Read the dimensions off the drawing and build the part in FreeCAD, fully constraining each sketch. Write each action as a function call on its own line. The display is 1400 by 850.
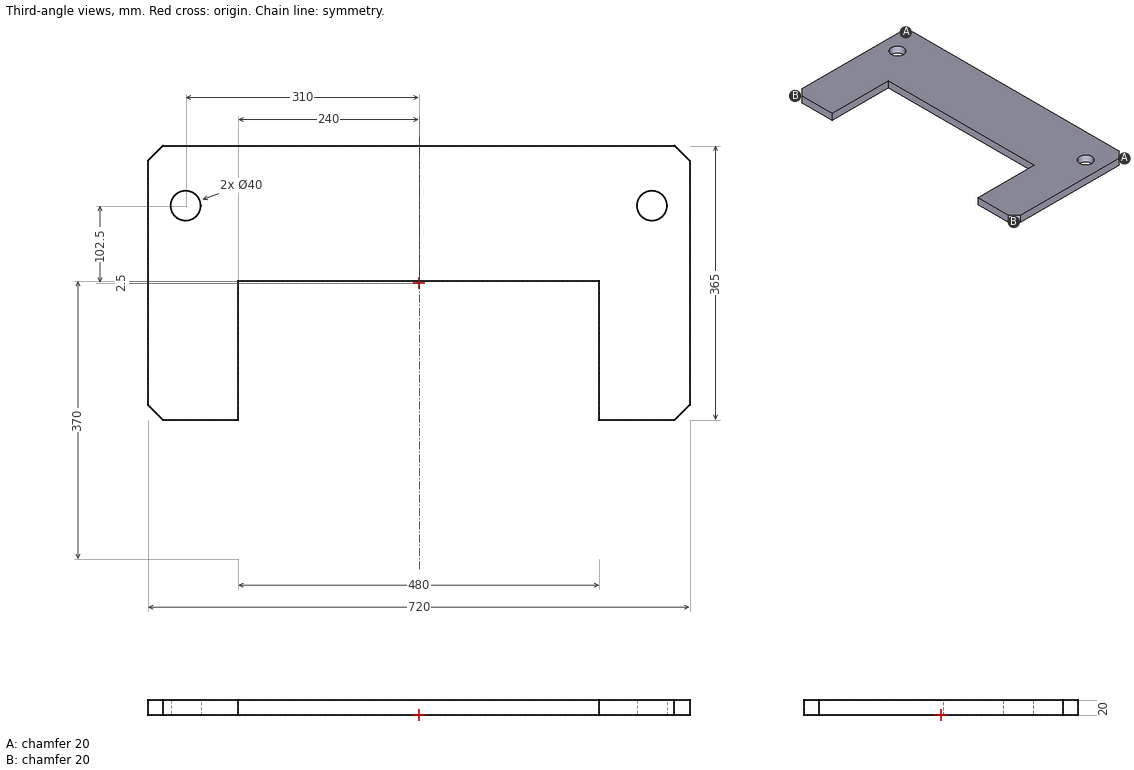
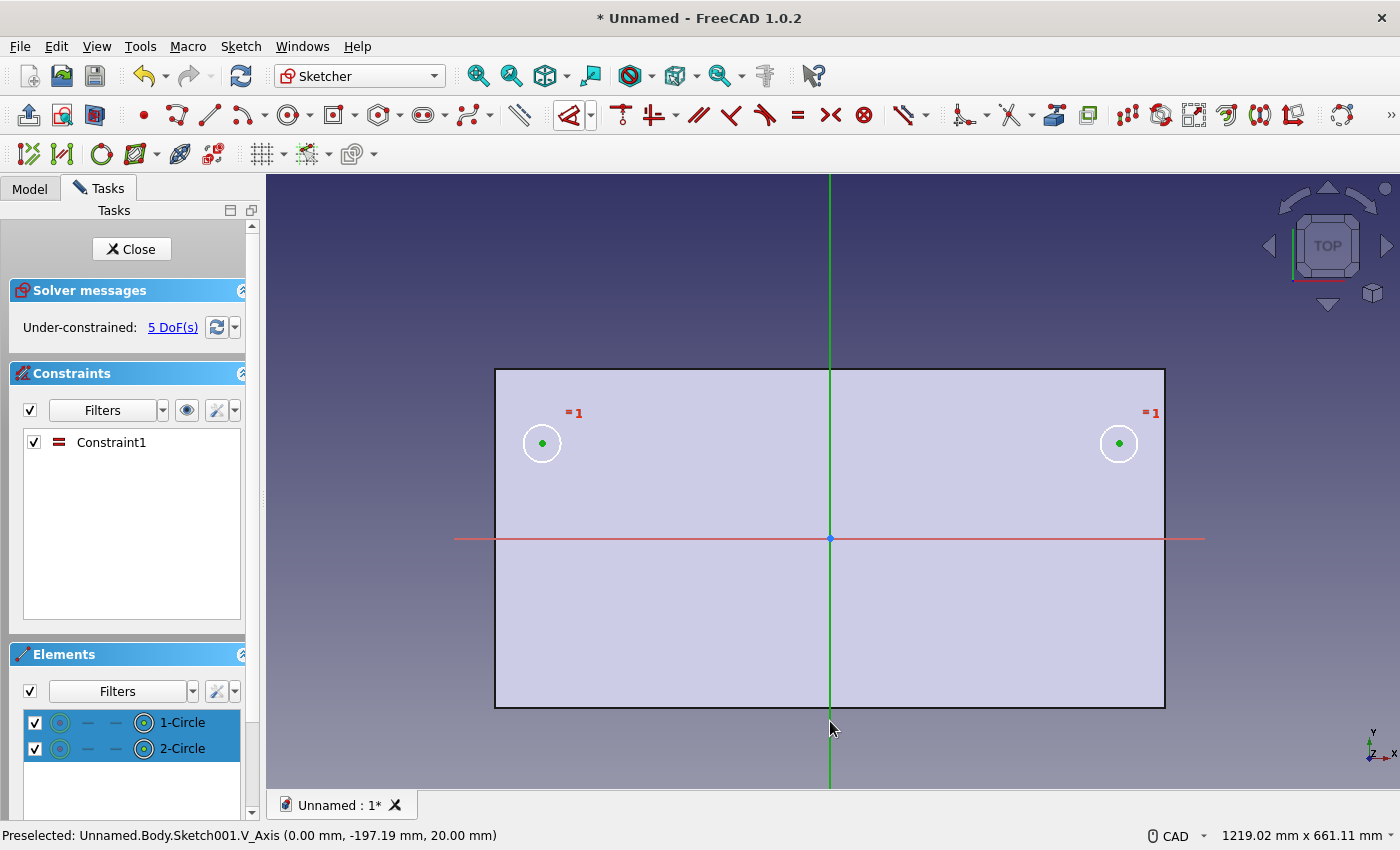
key(s)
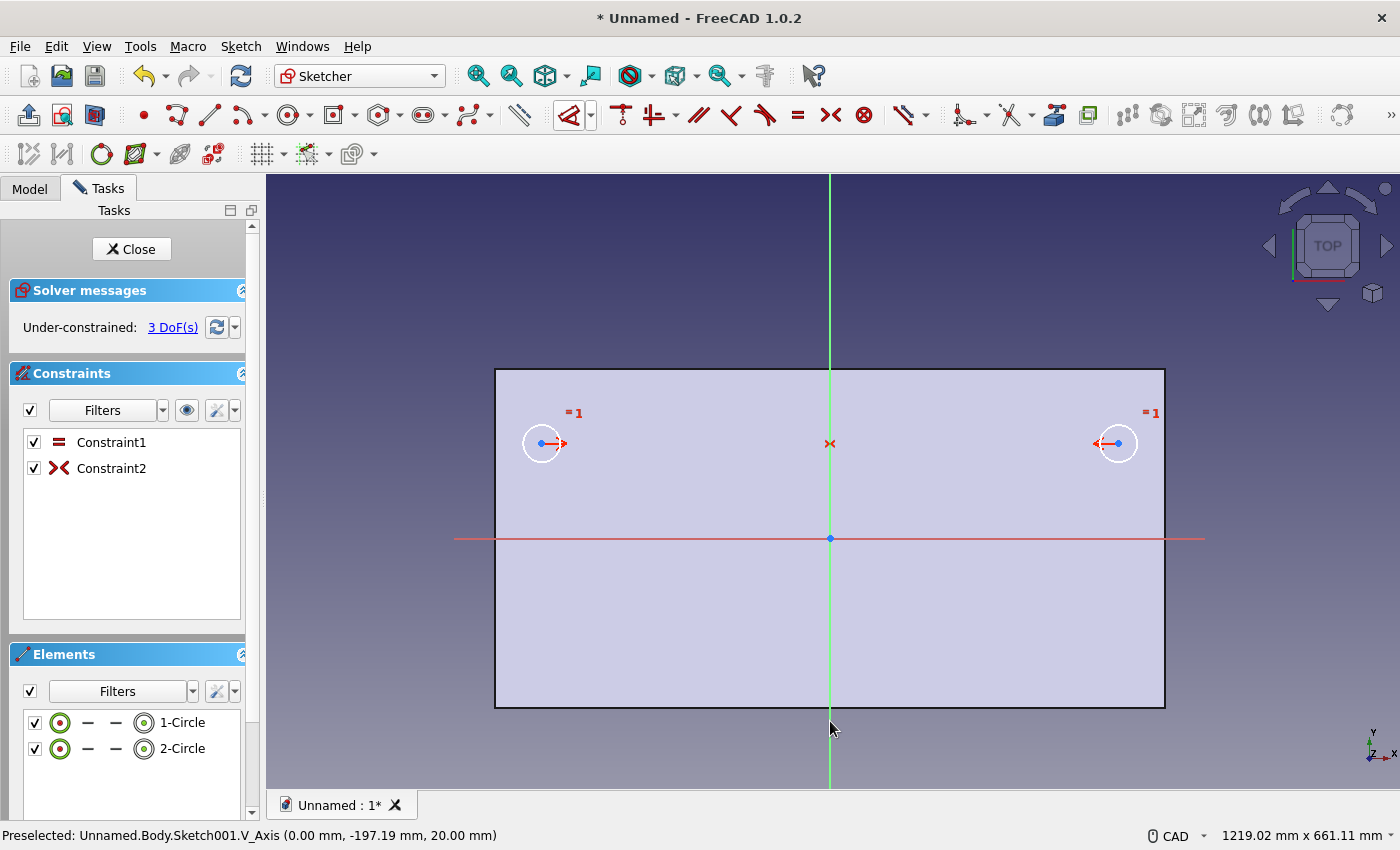
click(555, 431)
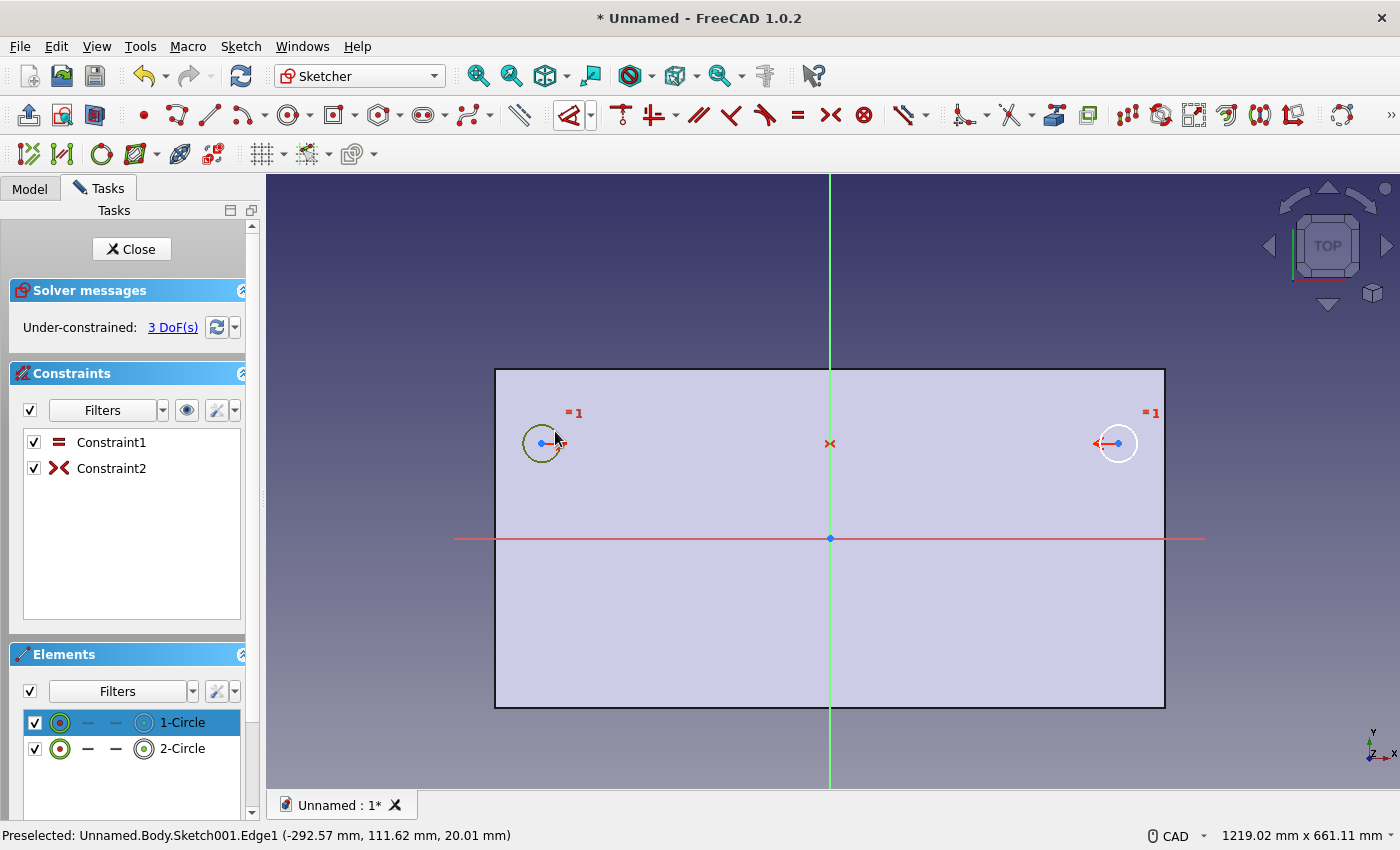
key(k)
key(o)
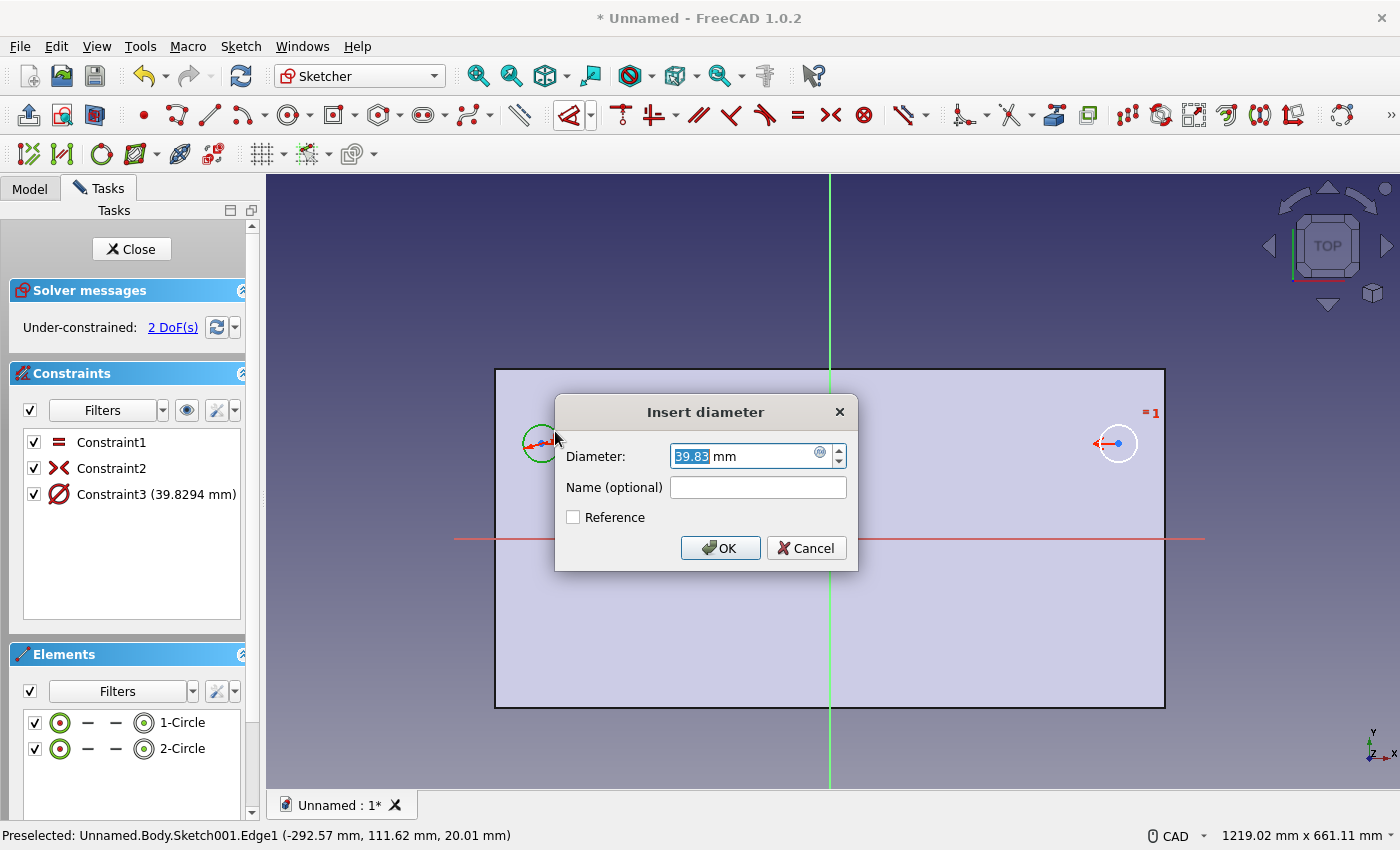
text(40)
key(Return)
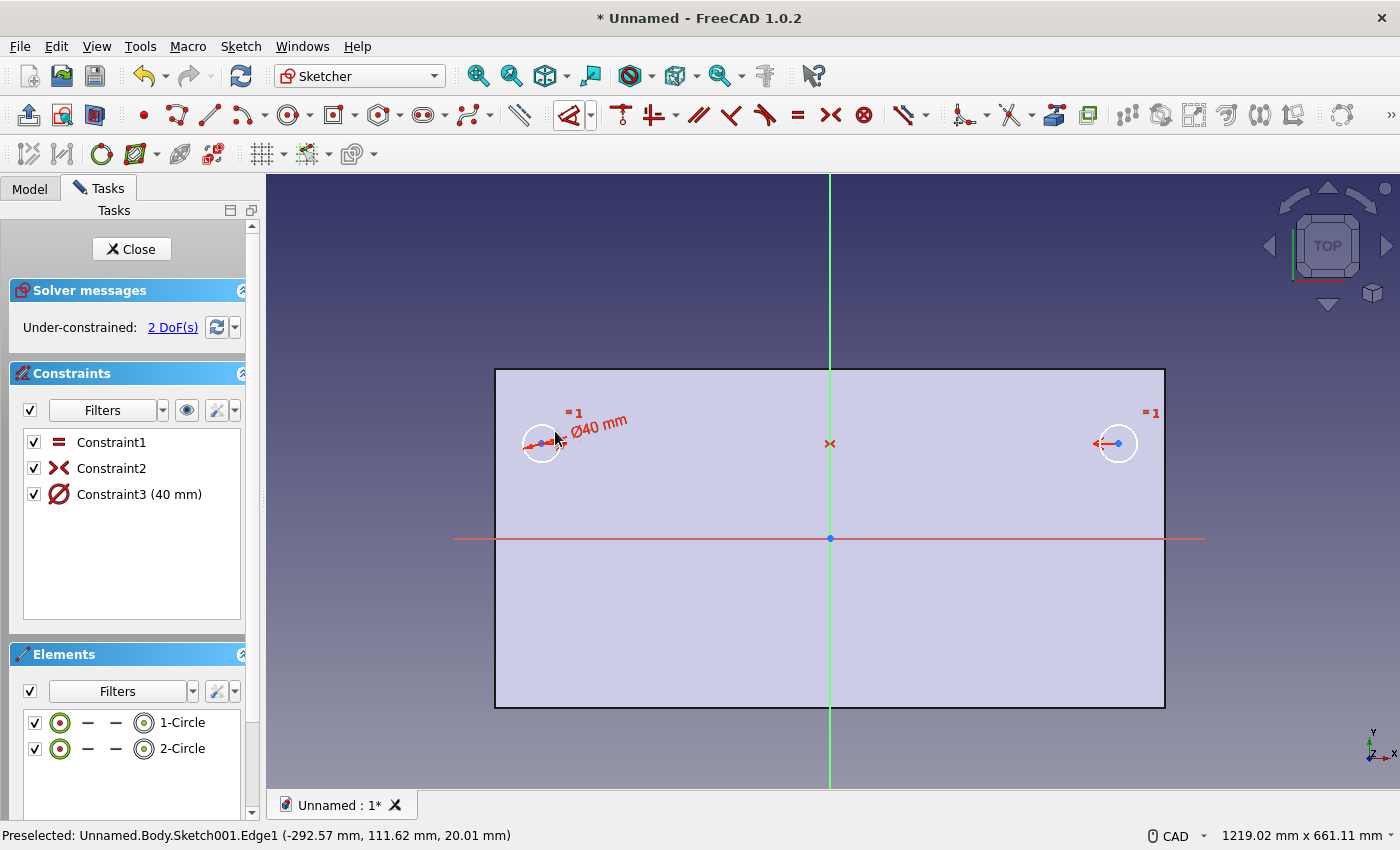
click(542, 444)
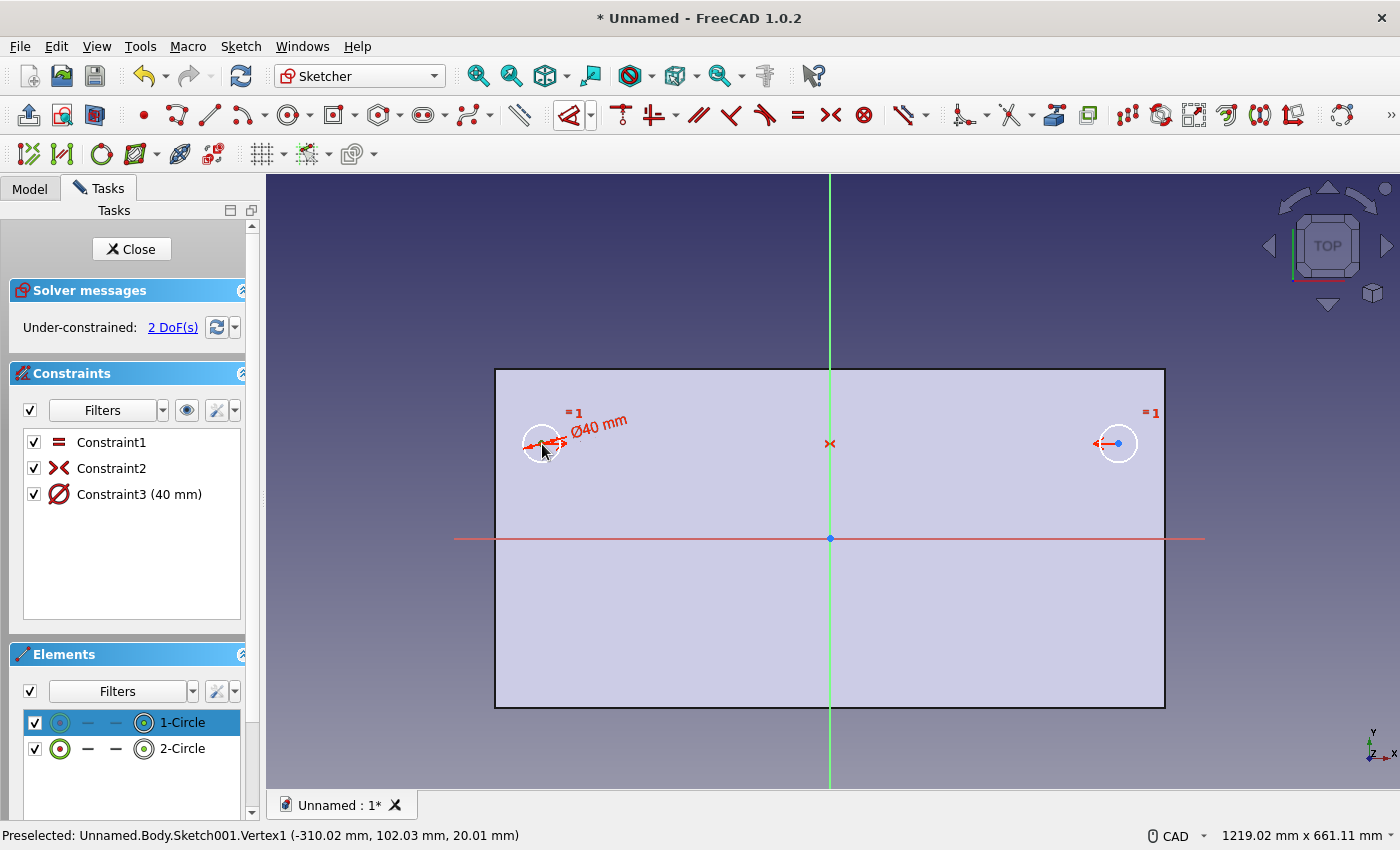
key(l)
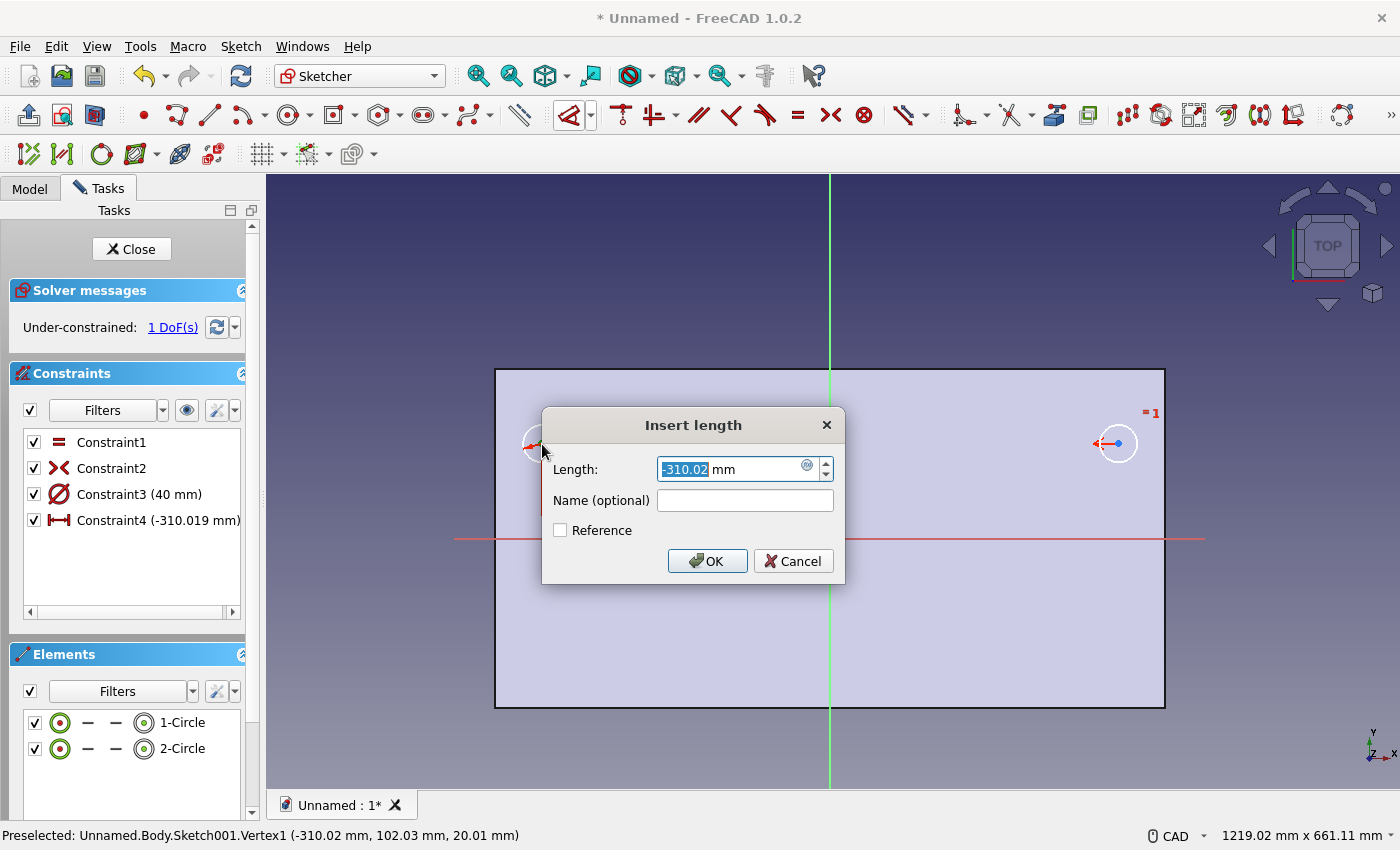
text(-310)
key(Return)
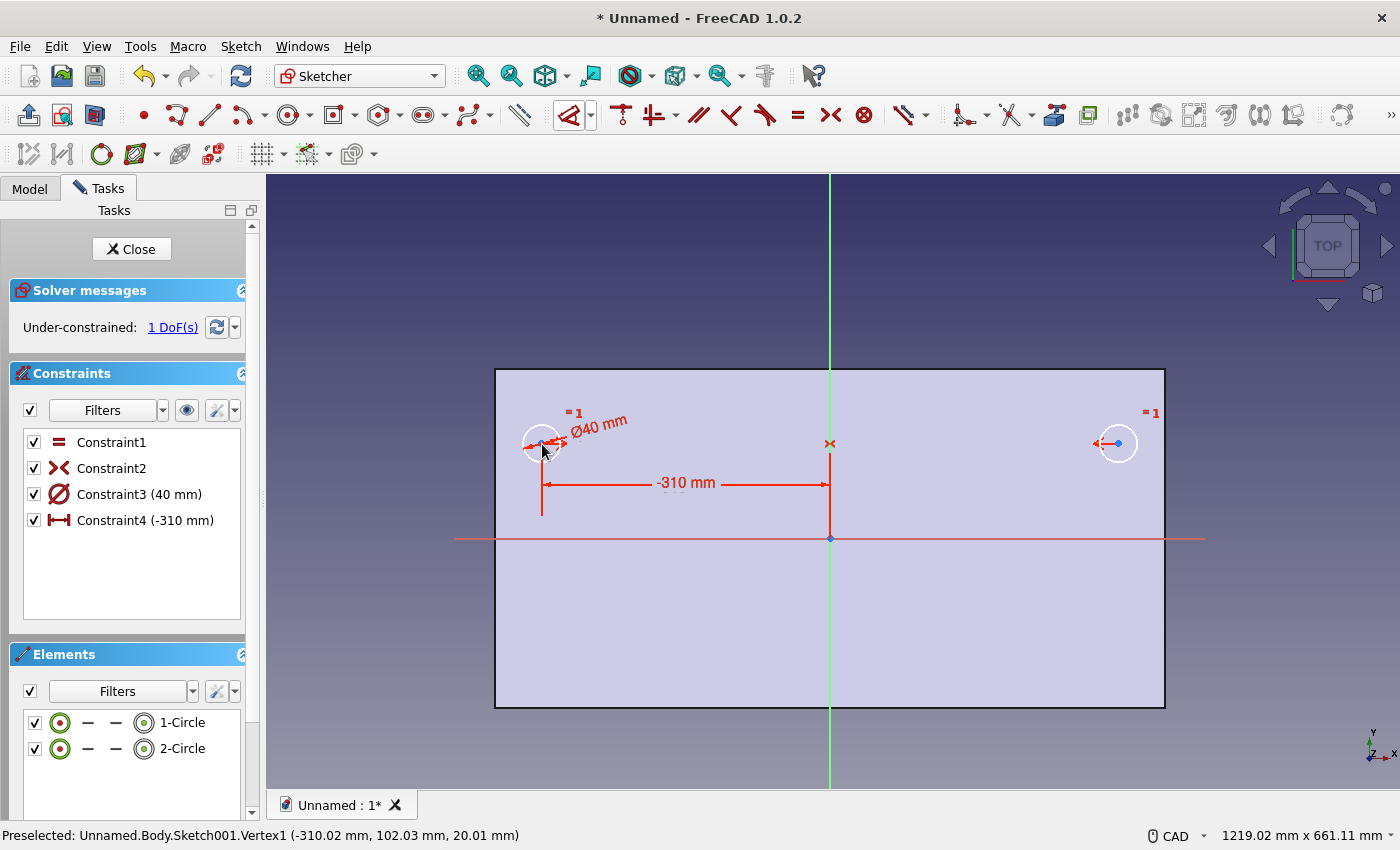
click(542, 444)